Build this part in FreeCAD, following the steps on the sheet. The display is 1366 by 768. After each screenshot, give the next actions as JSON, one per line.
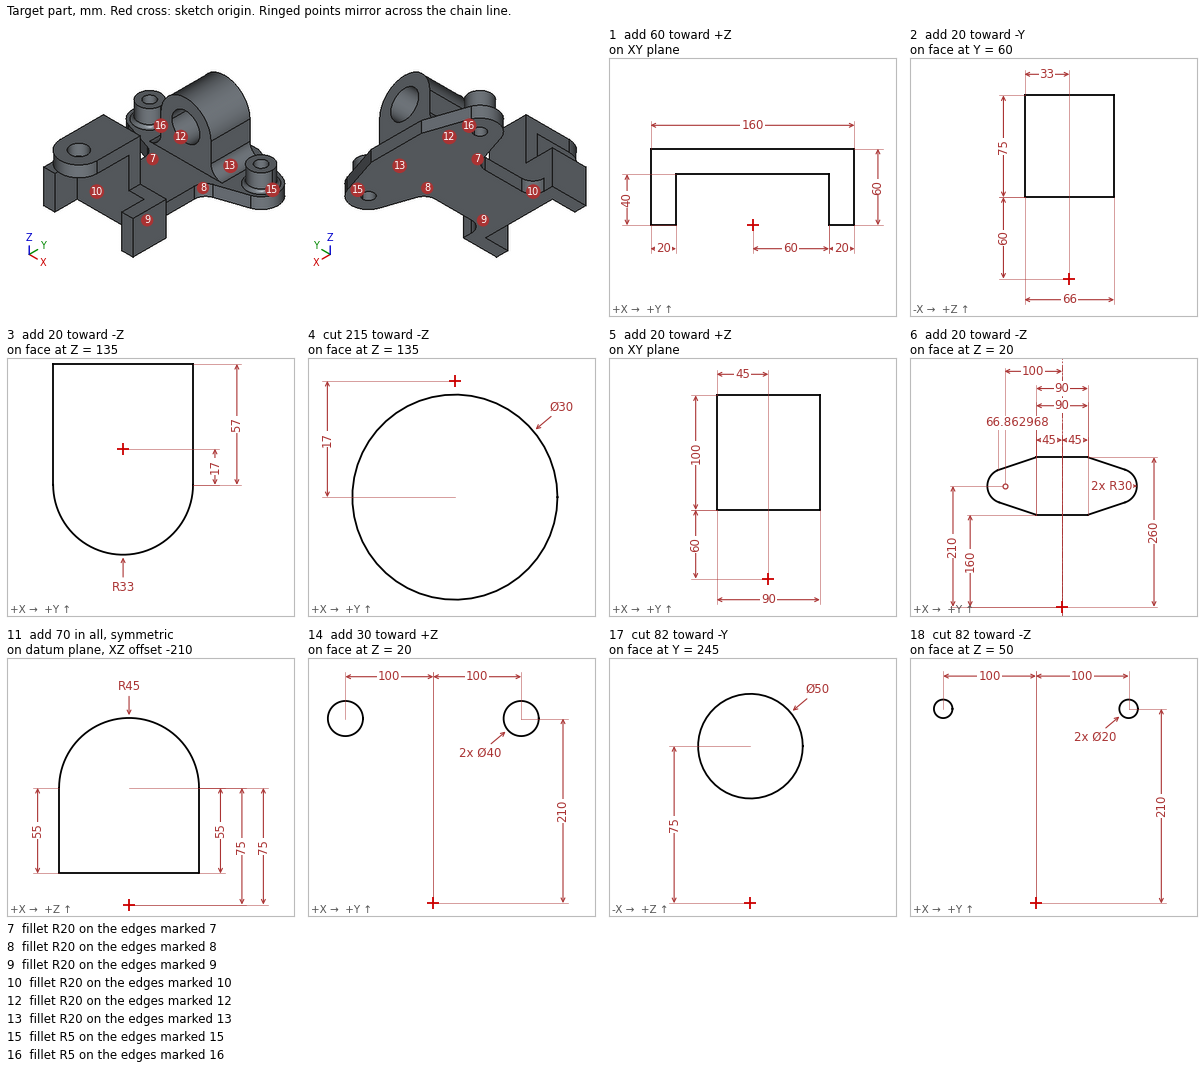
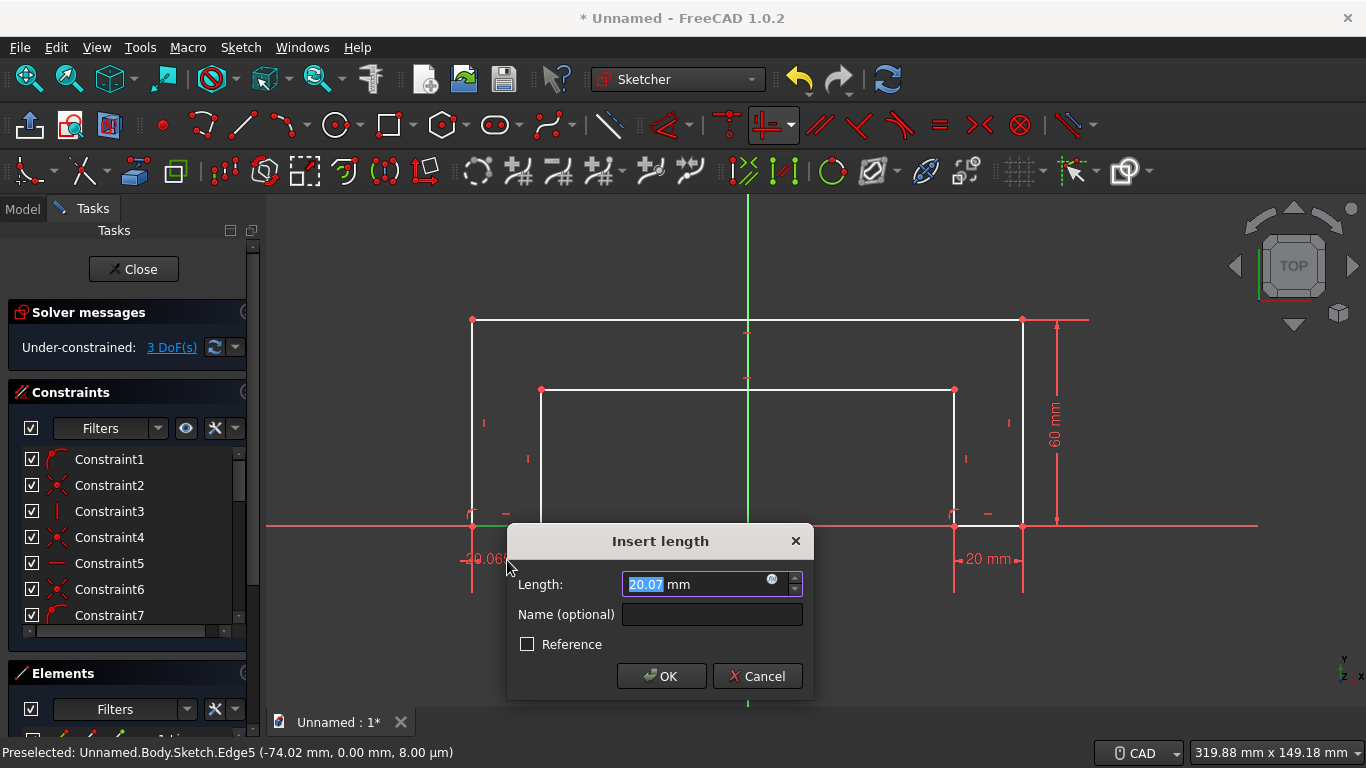
{"action": "type", "text": "20"}
{"action": "key", "text": "Return"}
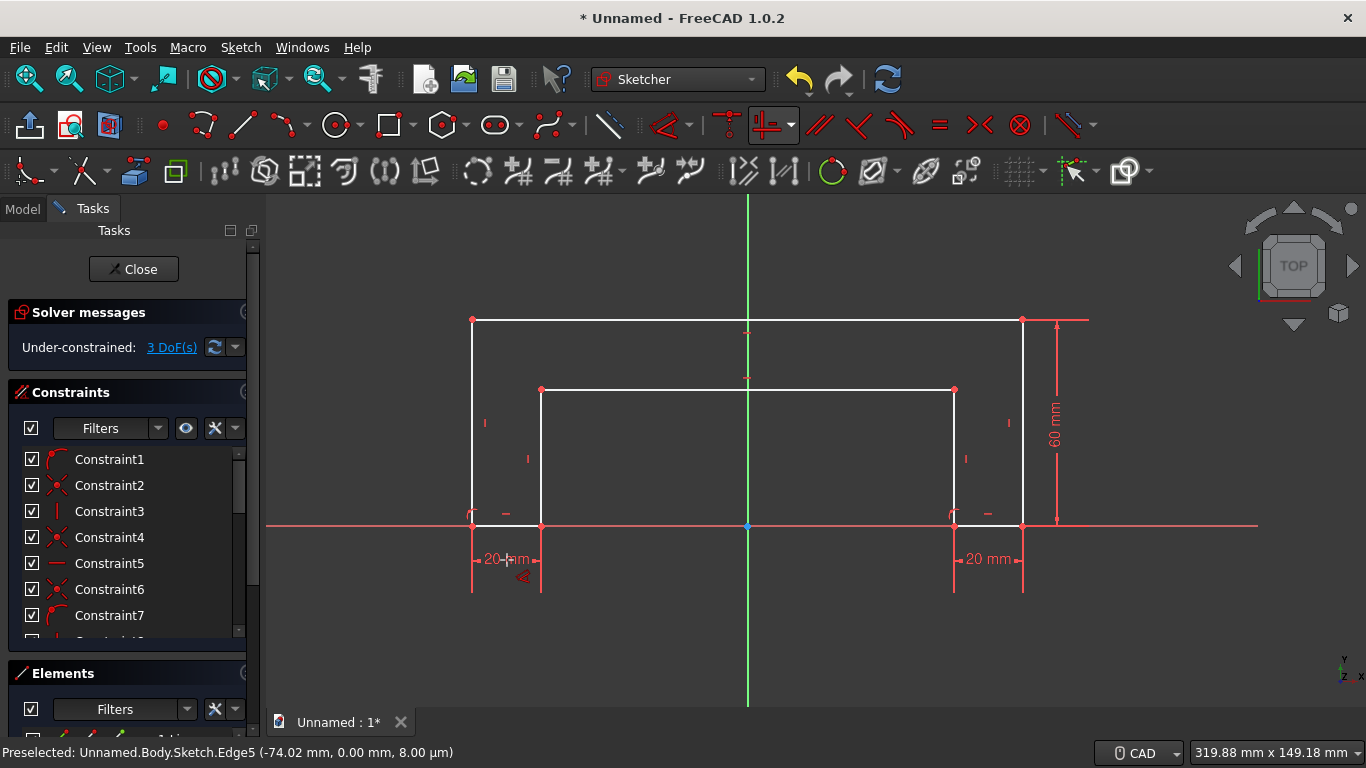
{"action": "left_click", "coordinate": [541, 485]}
{"action": "left_click", "coordinate": [507, 458]}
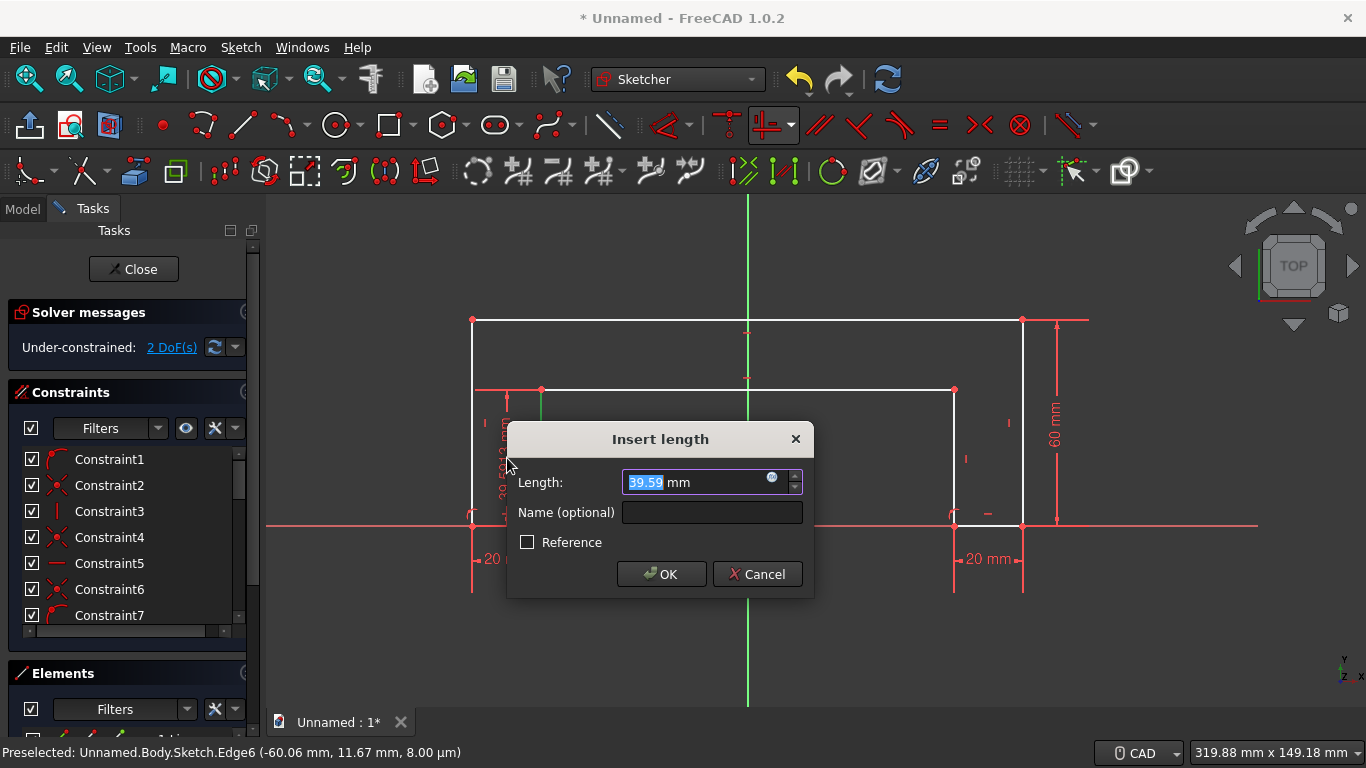
{"action": "type", "text": "40"}
{"action": "key", "text": "Return"}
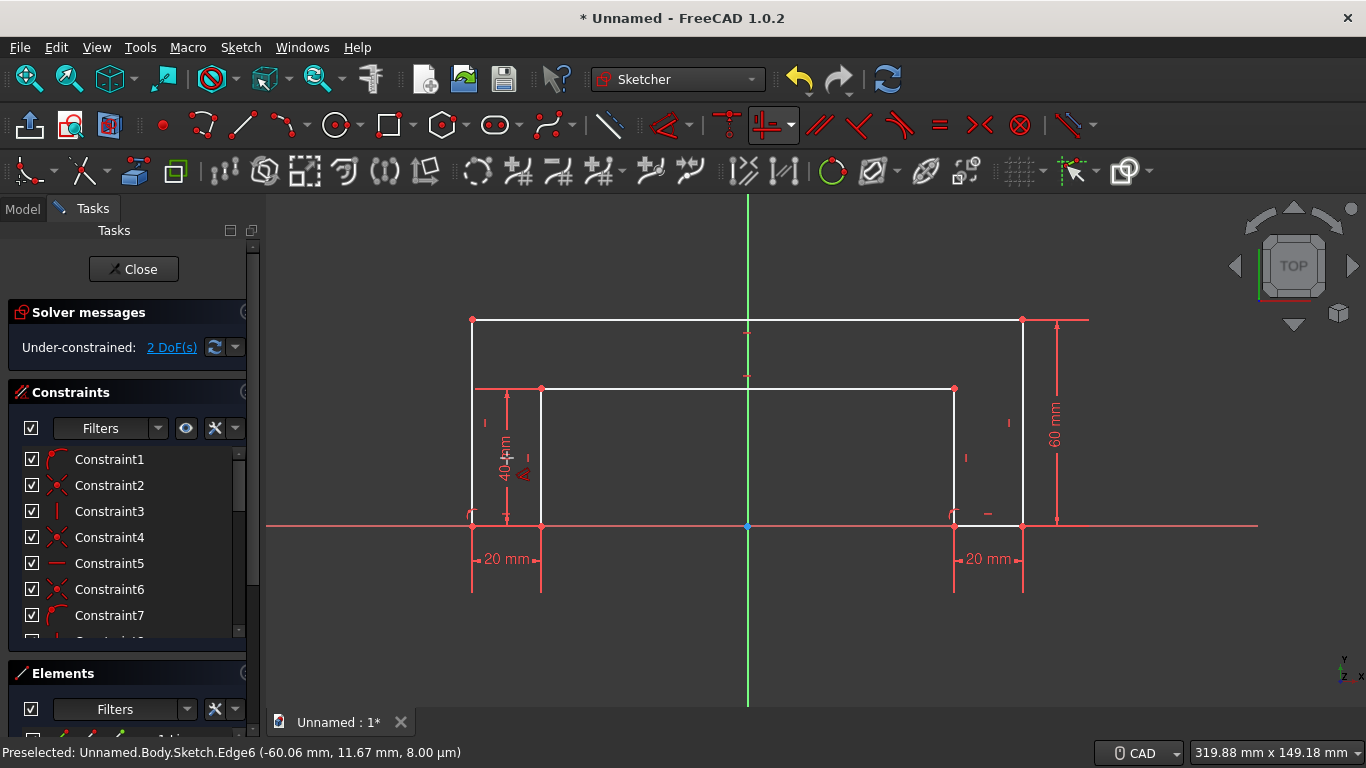
{"action": "left_click", "coordinate": [858, 320]}
{"action": "left_click", "coordinate": [621, 286]}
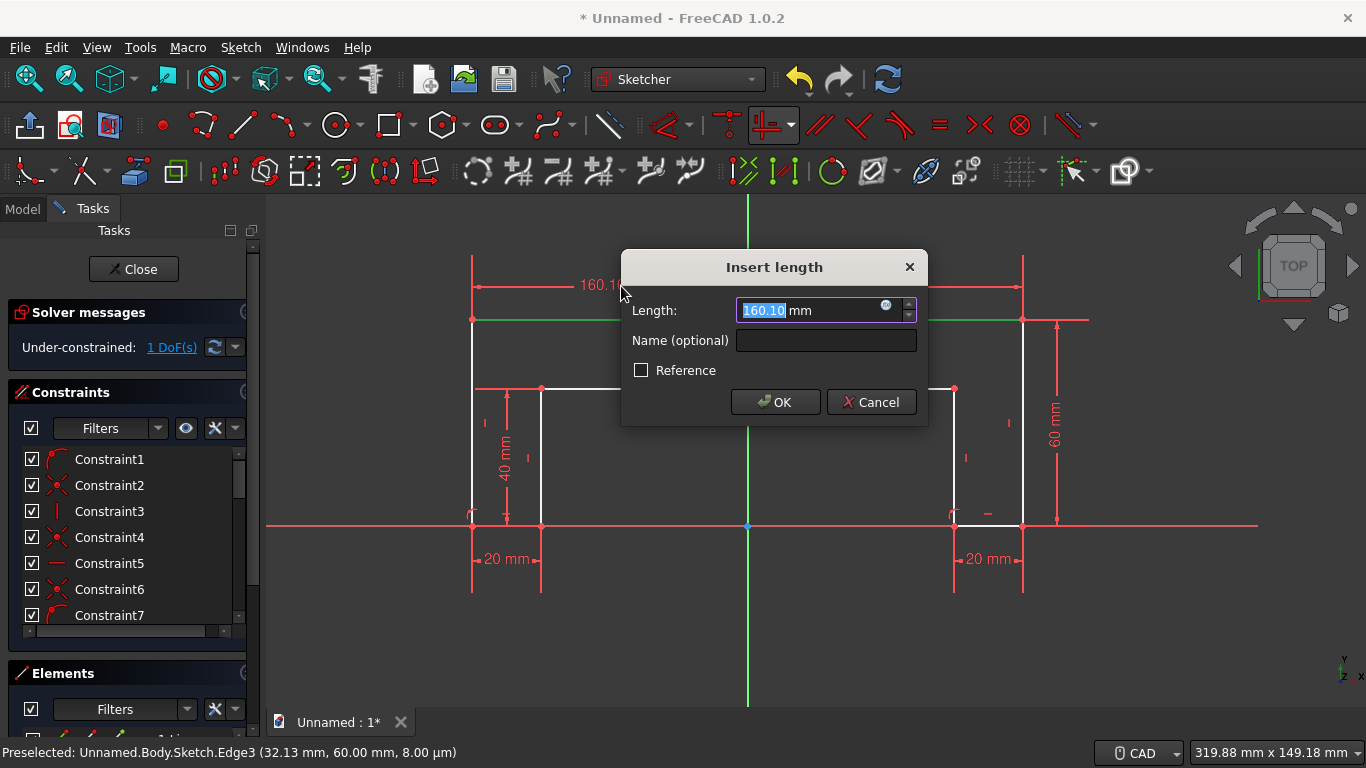
{"action": "type", "text": "160"}
{"action": "key", "text": "Return"}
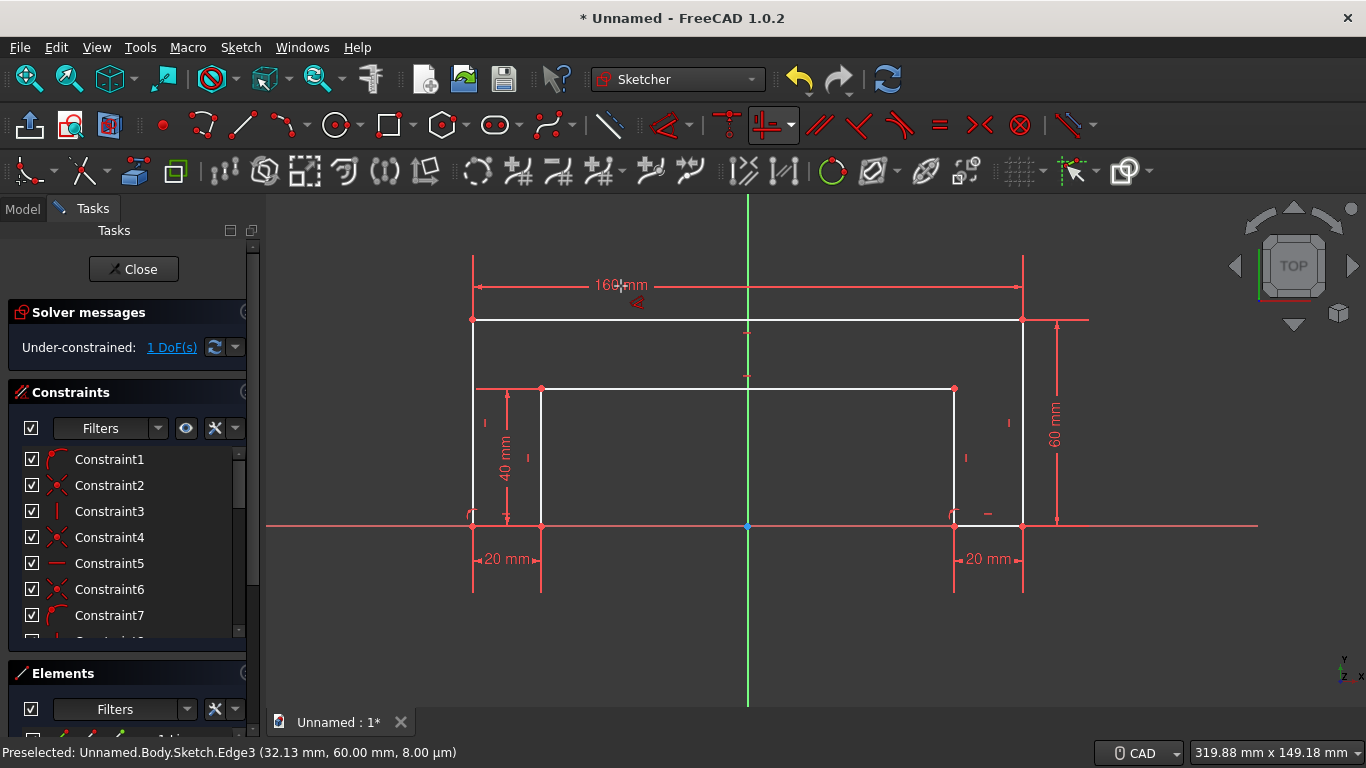
{"action": "left_click", "coordinate": [954, 526]}
{"action": "left_click", "coordinate": [851, 560]}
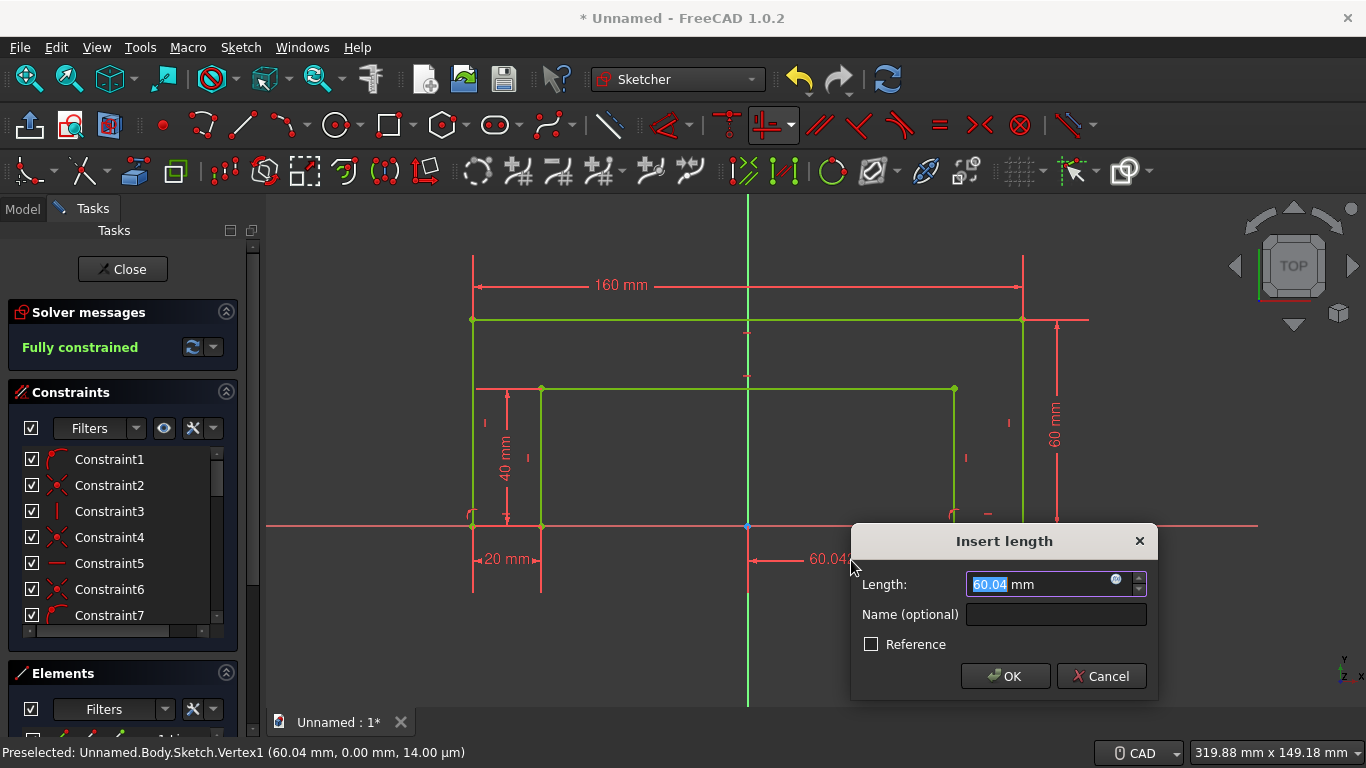
{"action": "type", "text": "60"}
{"action": "key", "text": "Return"}
{"action": "key", "text": "Escape"}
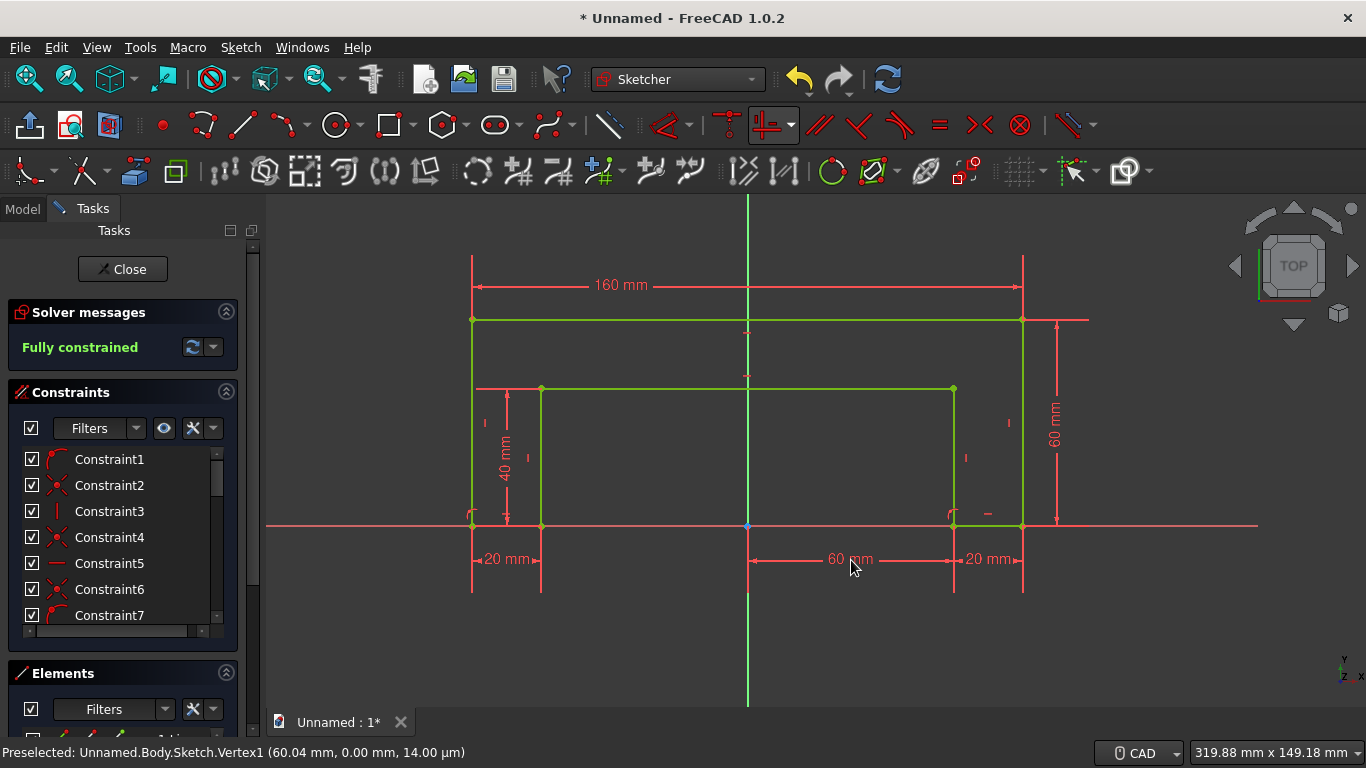
{"action": "left_click", "coordinate": [123, 269]}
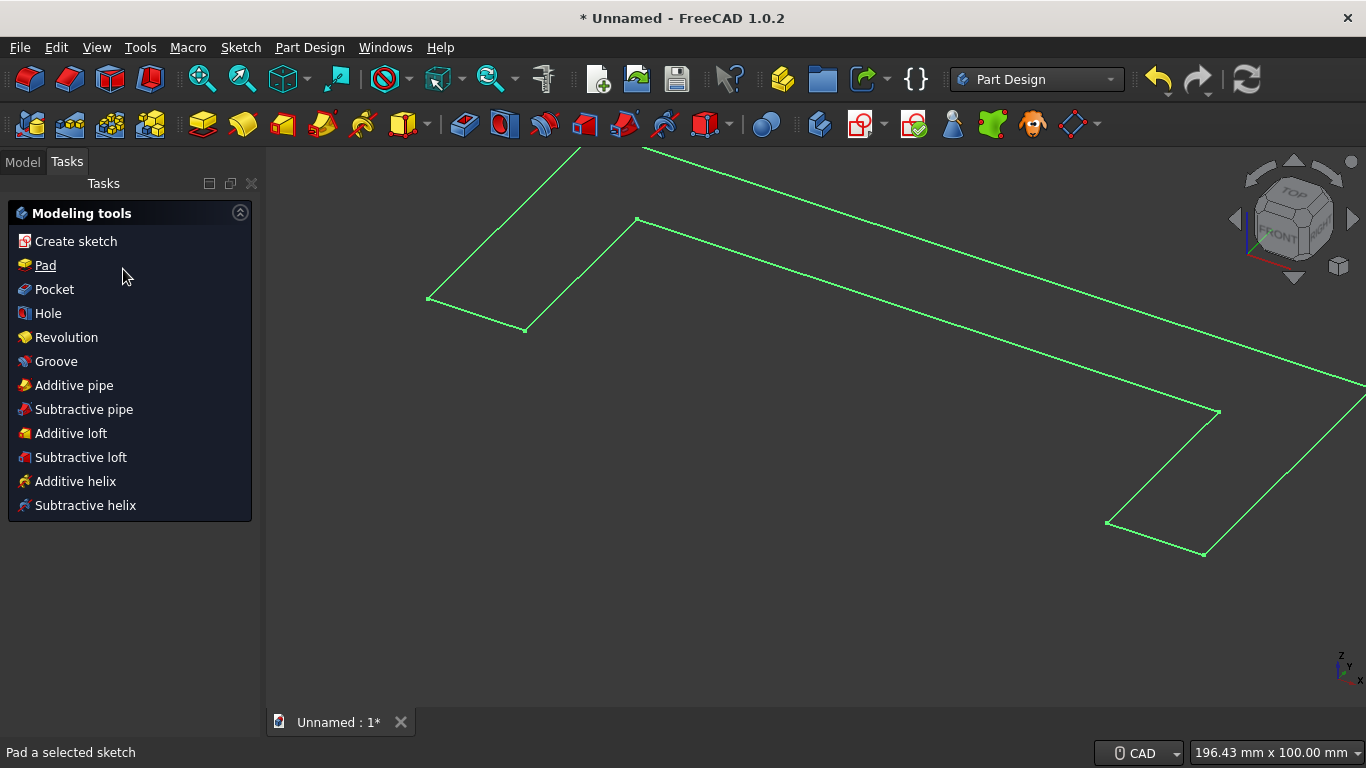
{"action": "left_click", "coordinate": [204, 124]}